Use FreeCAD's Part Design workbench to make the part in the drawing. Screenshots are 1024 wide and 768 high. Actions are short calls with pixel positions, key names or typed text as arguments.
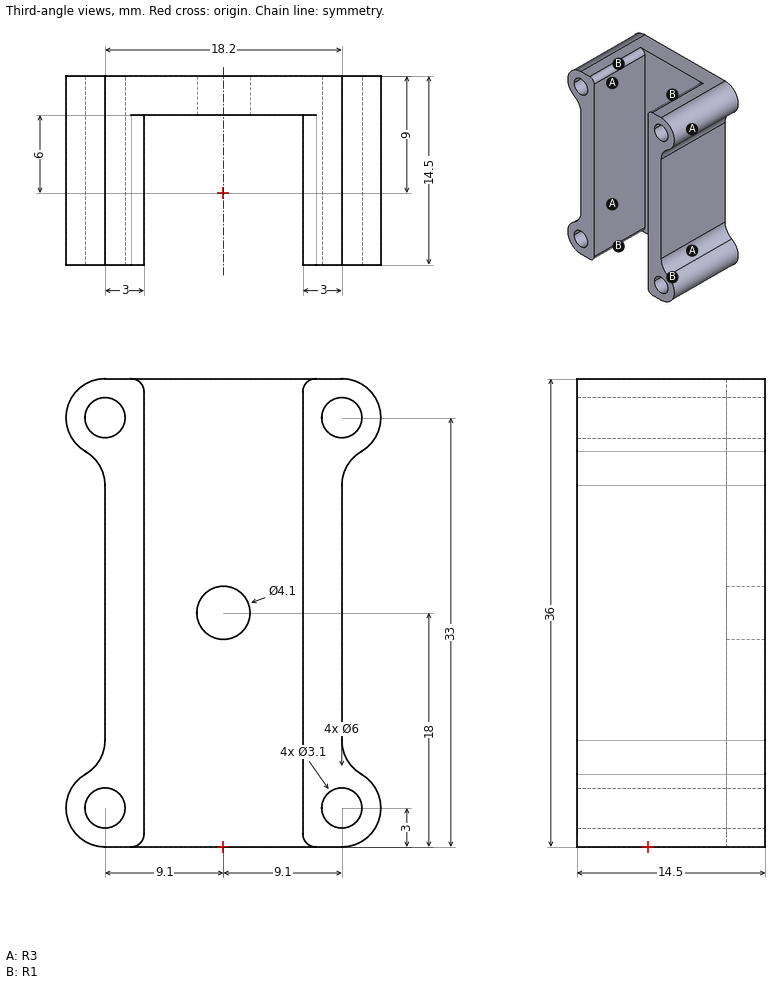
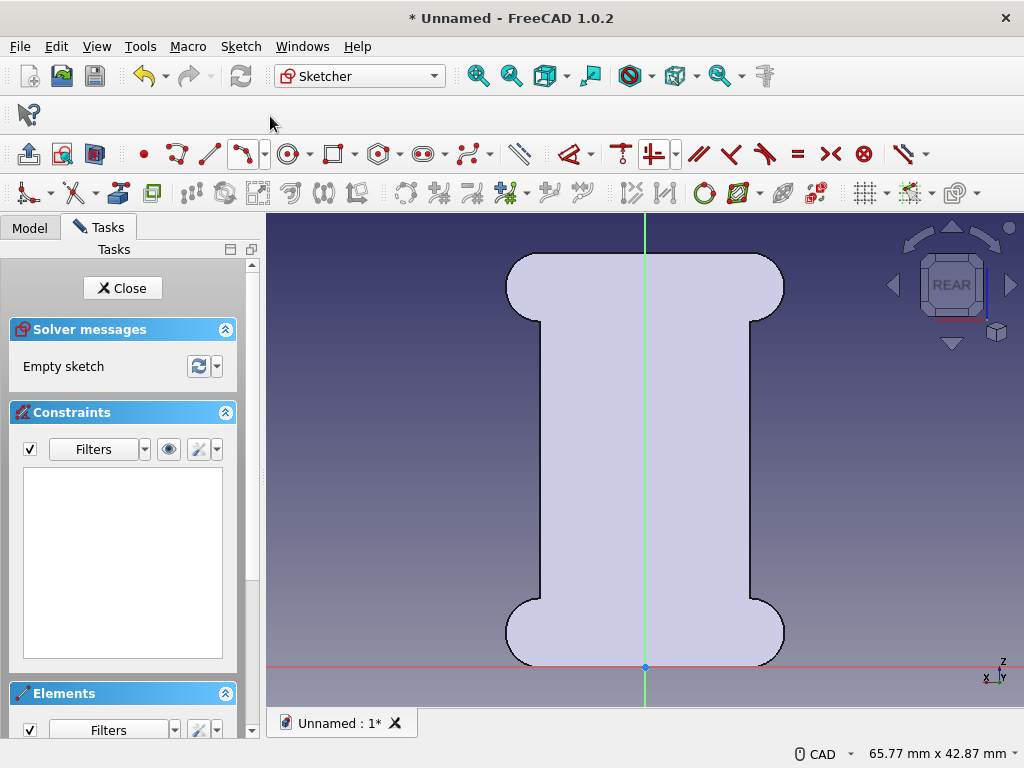
scroll(294, 422, down, 1)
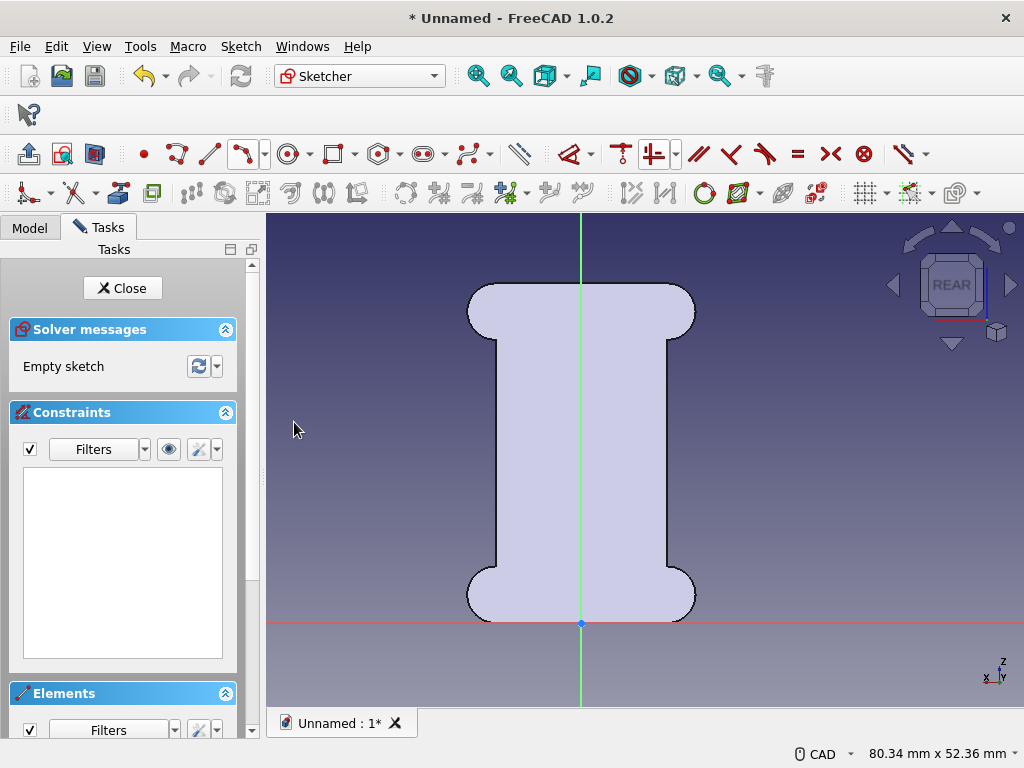
click(288, 154)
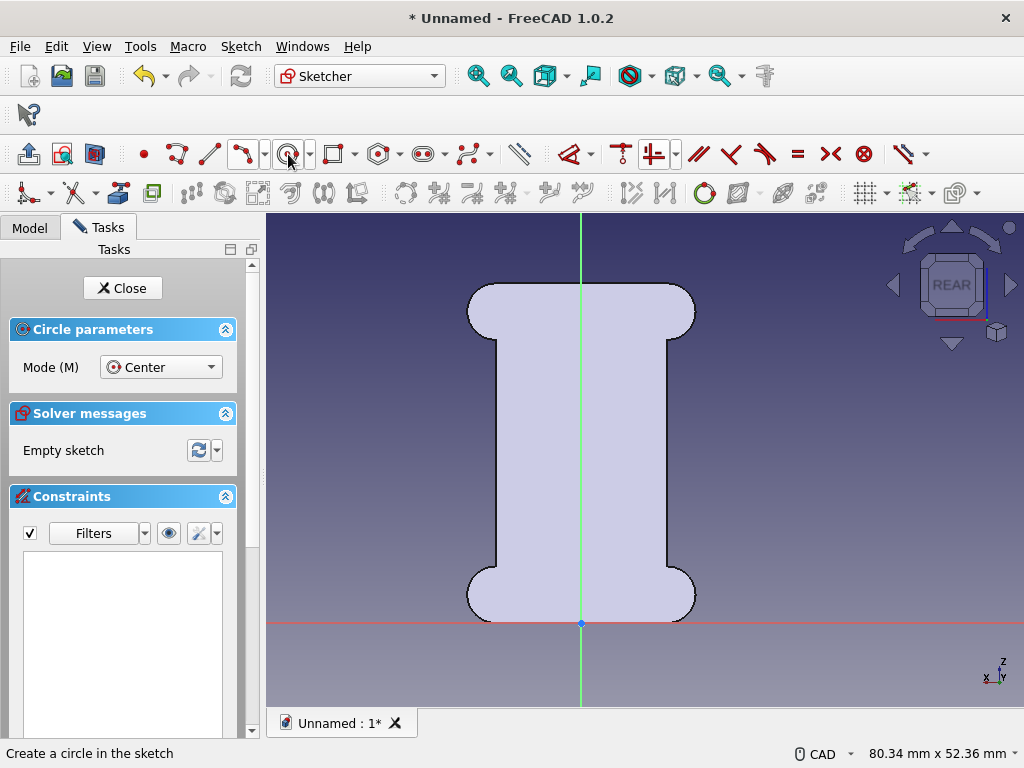
scroll(496, 595, up, 3)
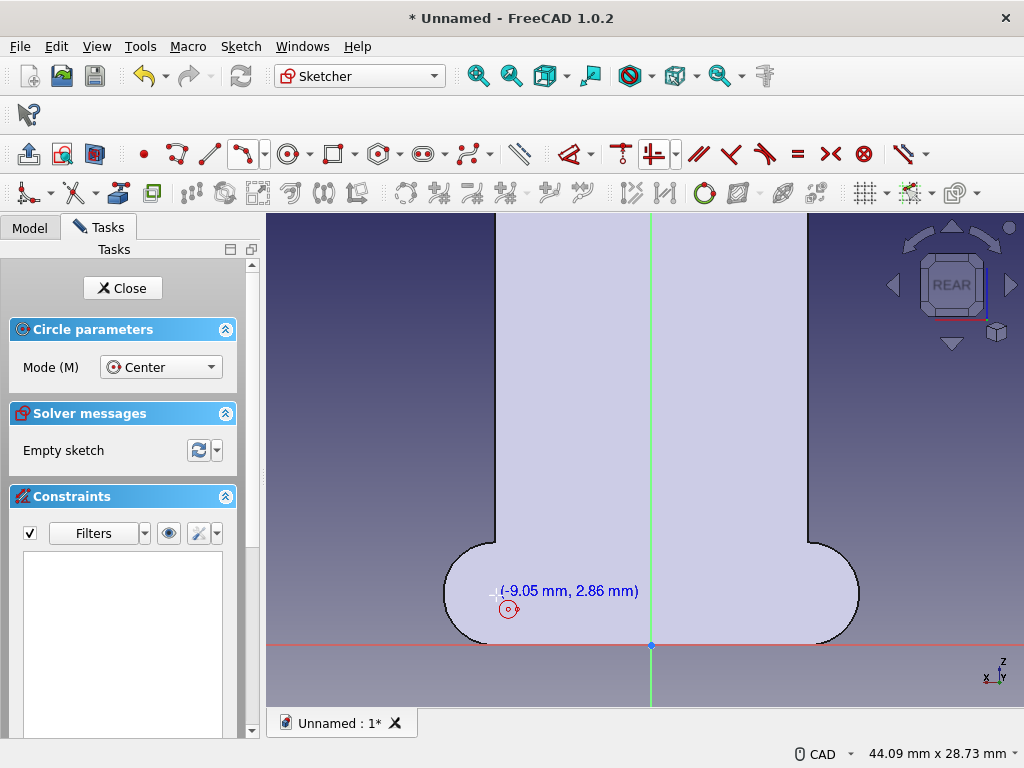
click(495, 594)
click(514, 575)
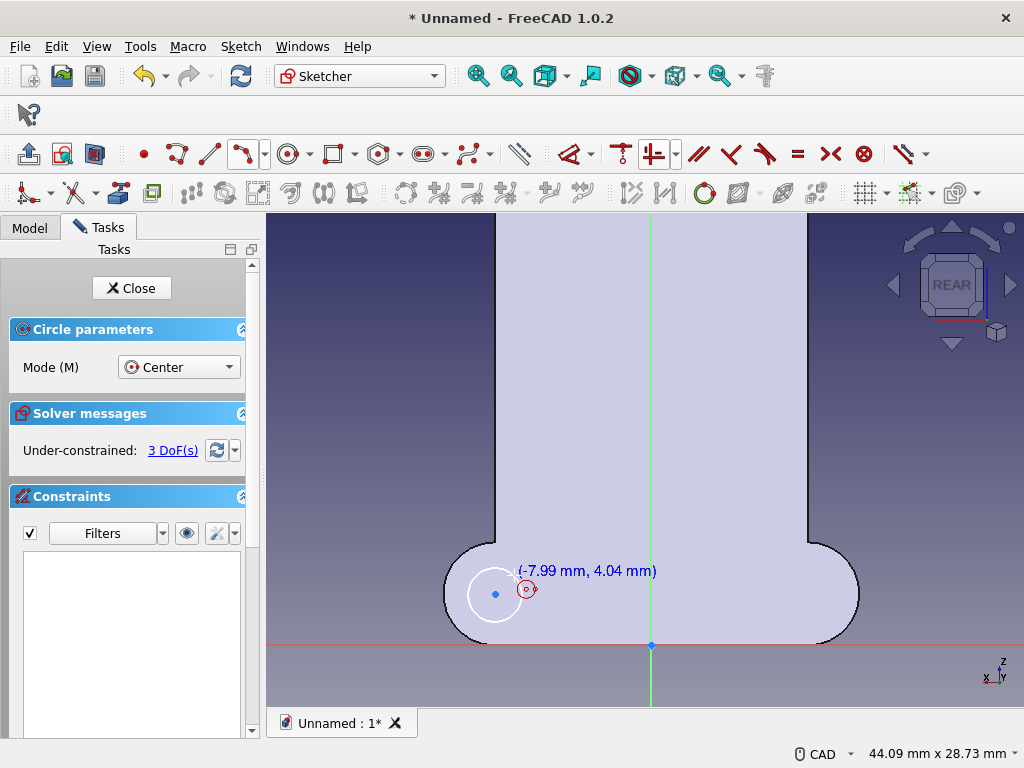
scroll(485, 596, down, 3)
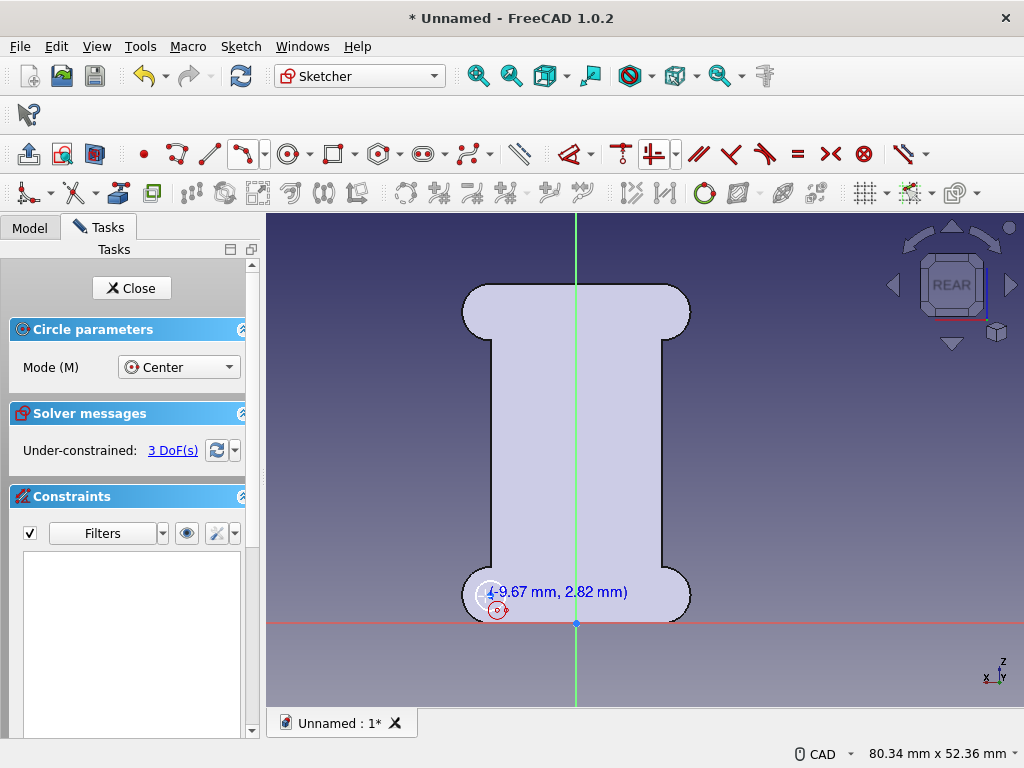
scroll(662, 312, up, 3)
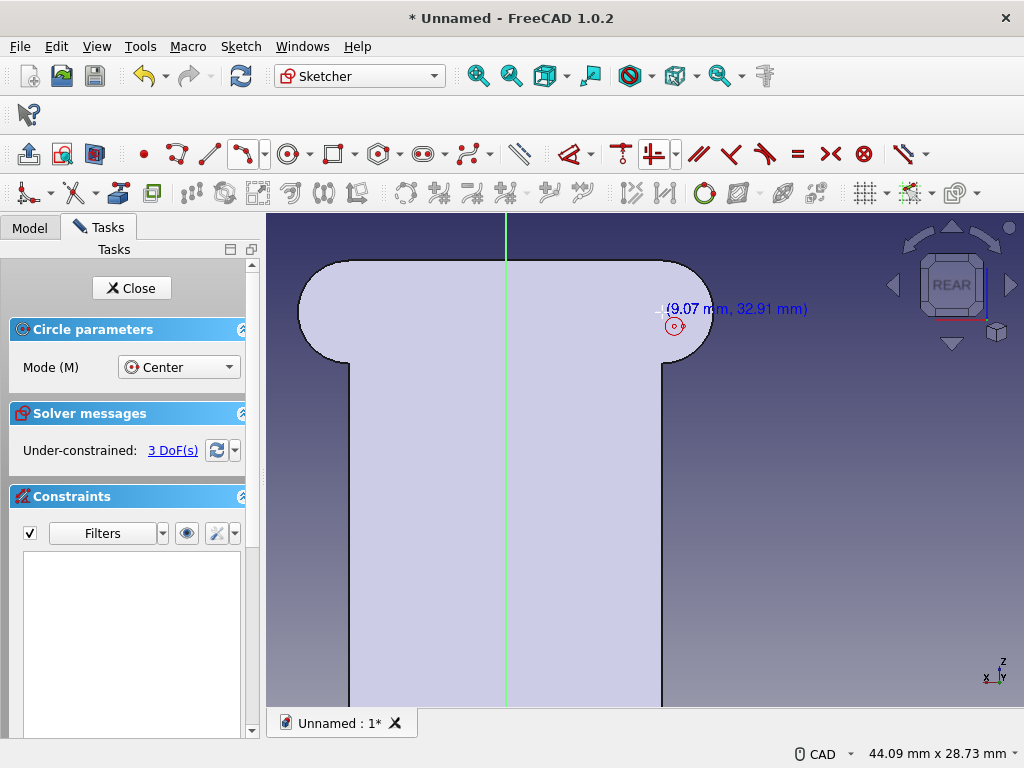
click(662, 312)
click(681, 293)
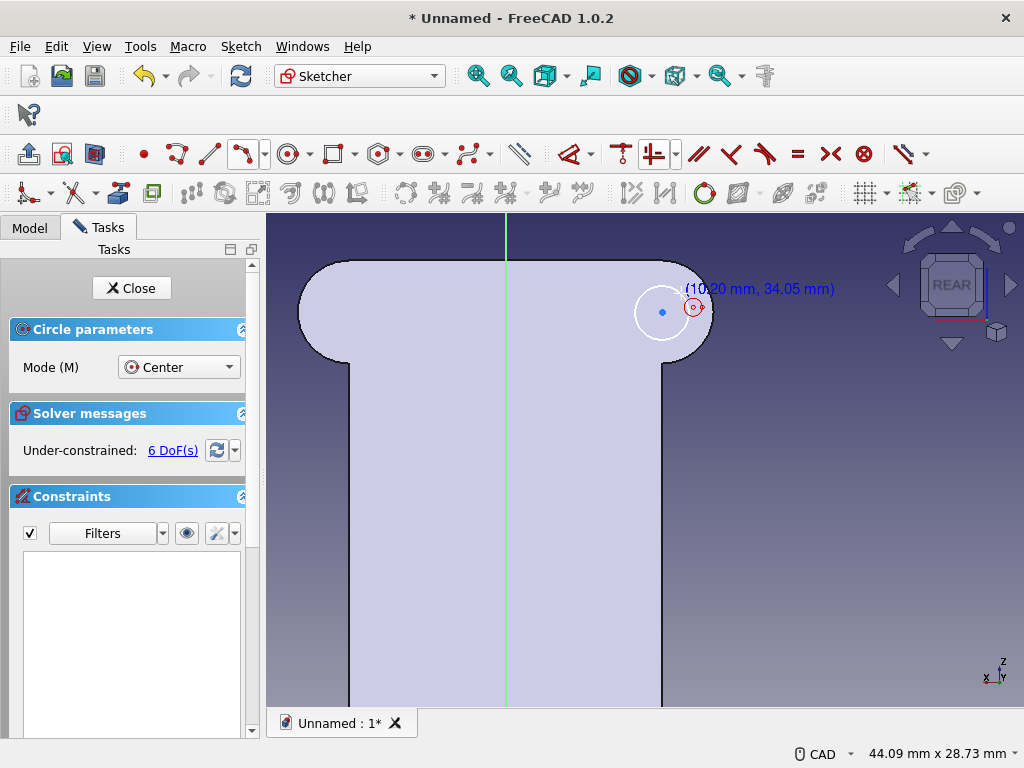
click(349, 312)
click(368, 293)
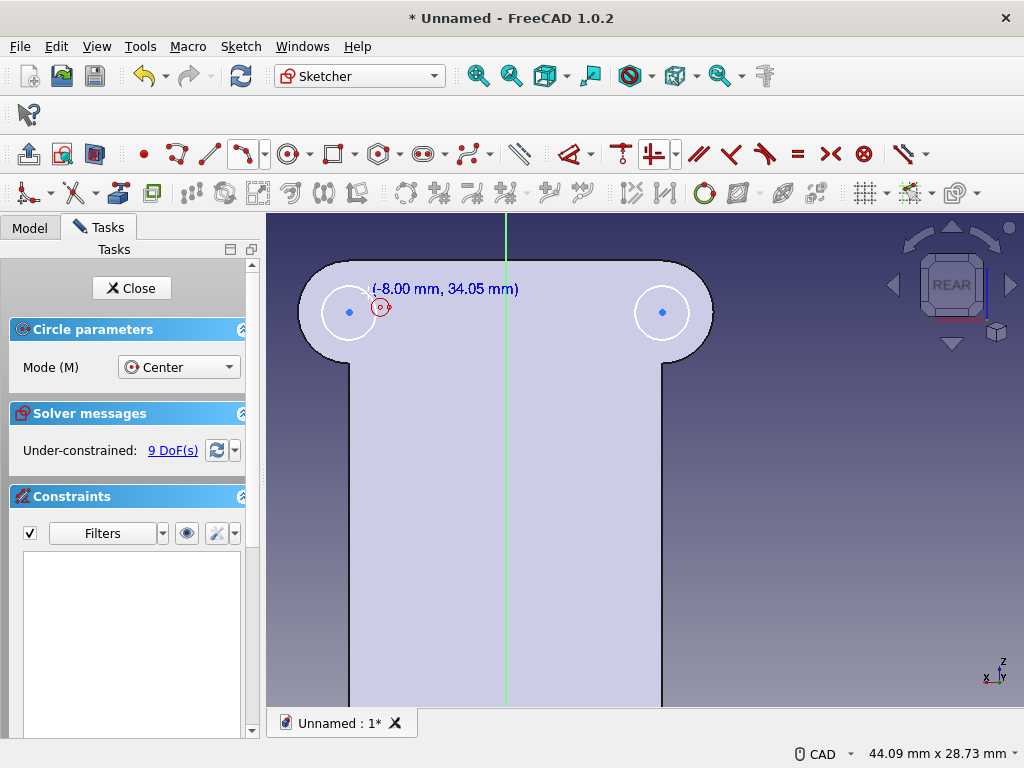
scroll(663, 311, down, 3)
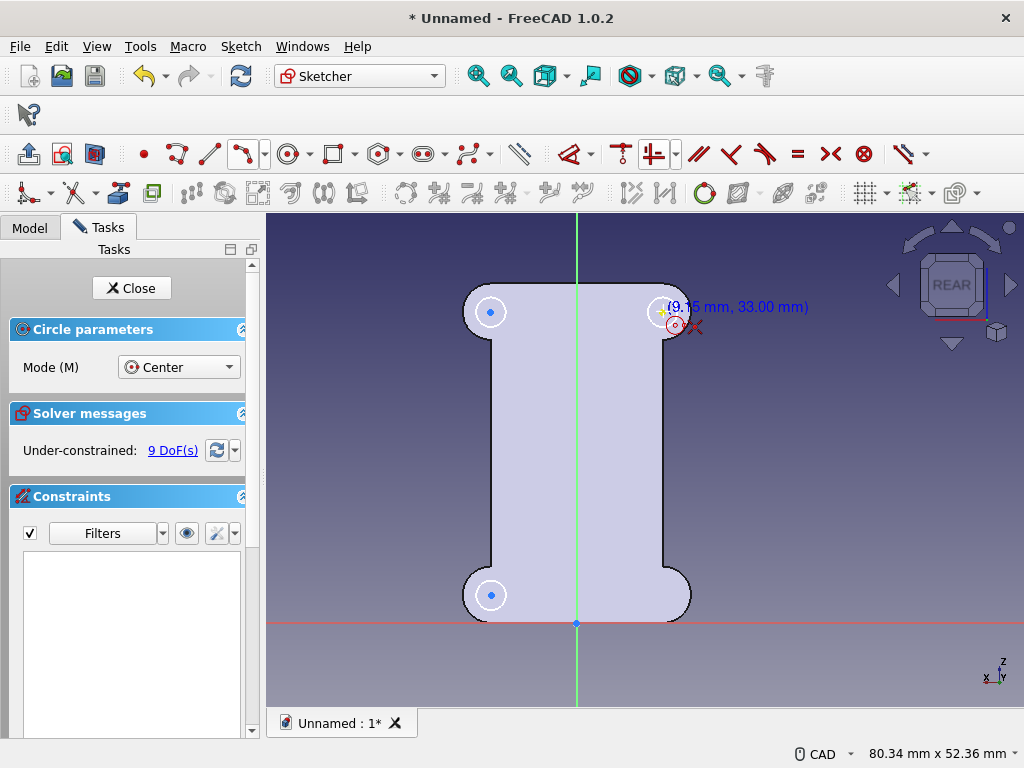
scroll(663, 595, up, 3)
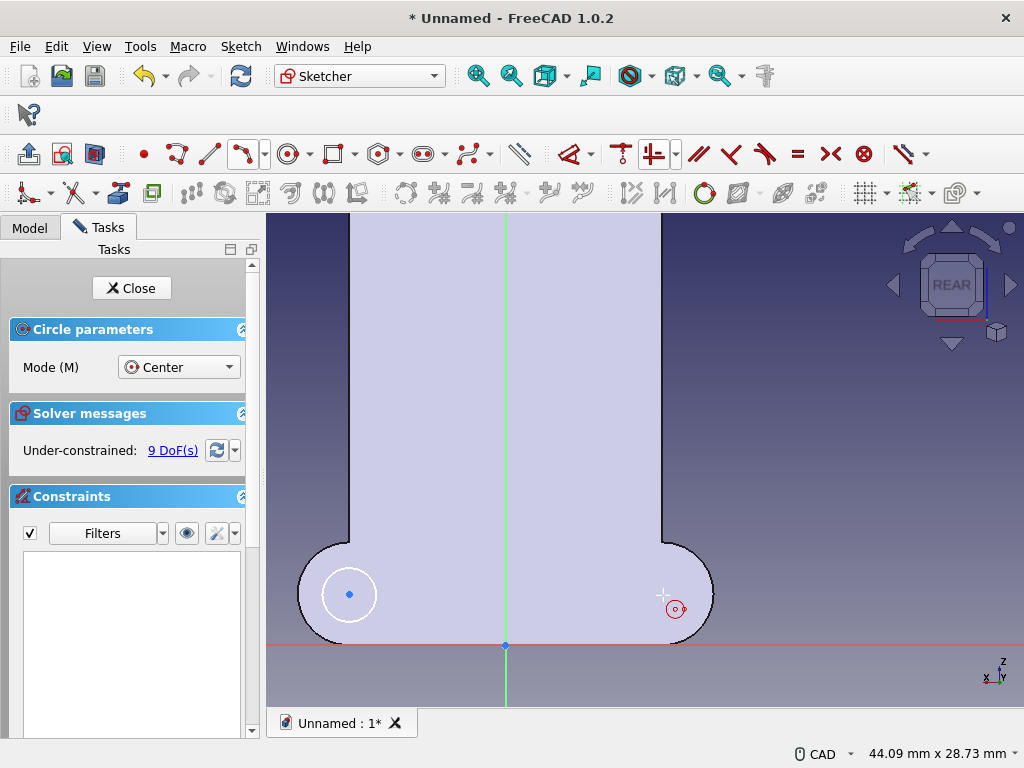
click(662, 594)
click(681, 575)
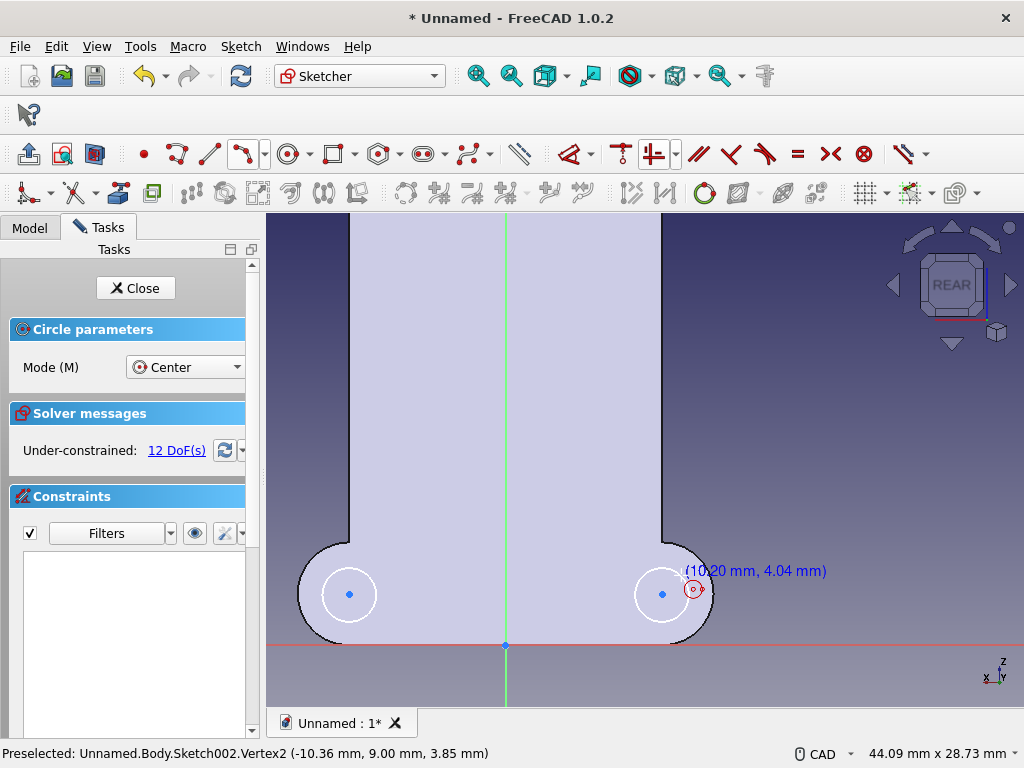
click(506, 336)
click(531, 311)
key(Escape)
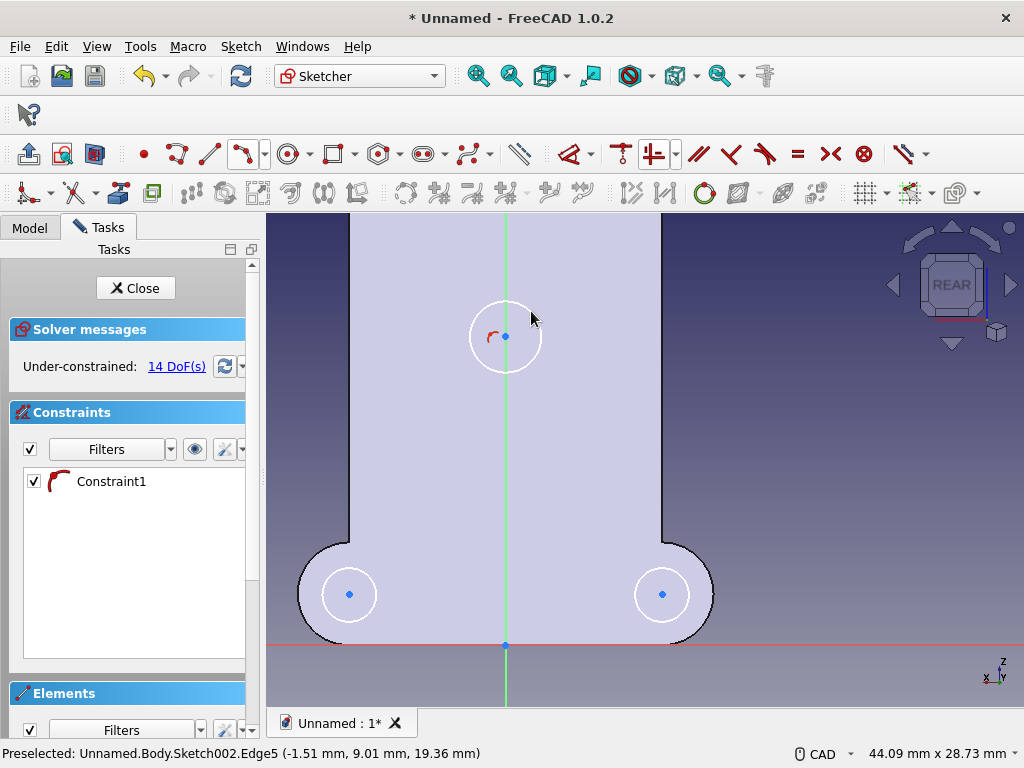
click(368, 576)